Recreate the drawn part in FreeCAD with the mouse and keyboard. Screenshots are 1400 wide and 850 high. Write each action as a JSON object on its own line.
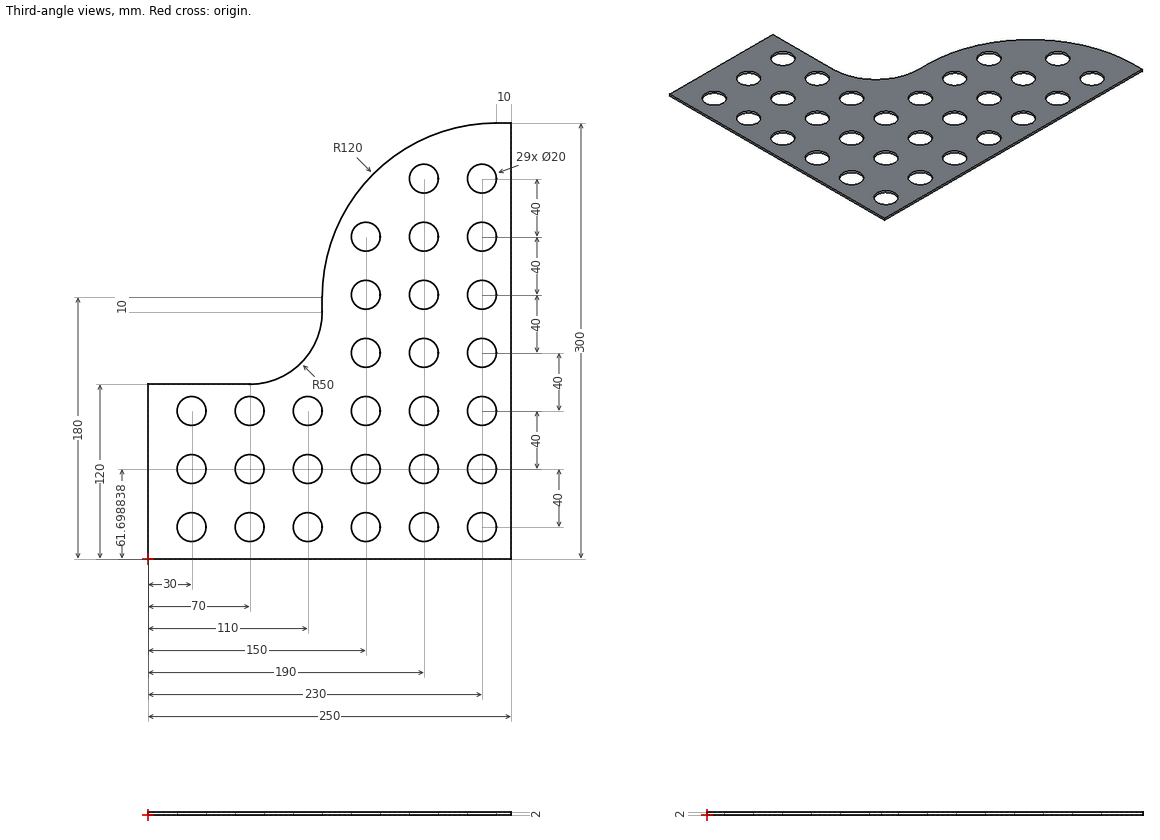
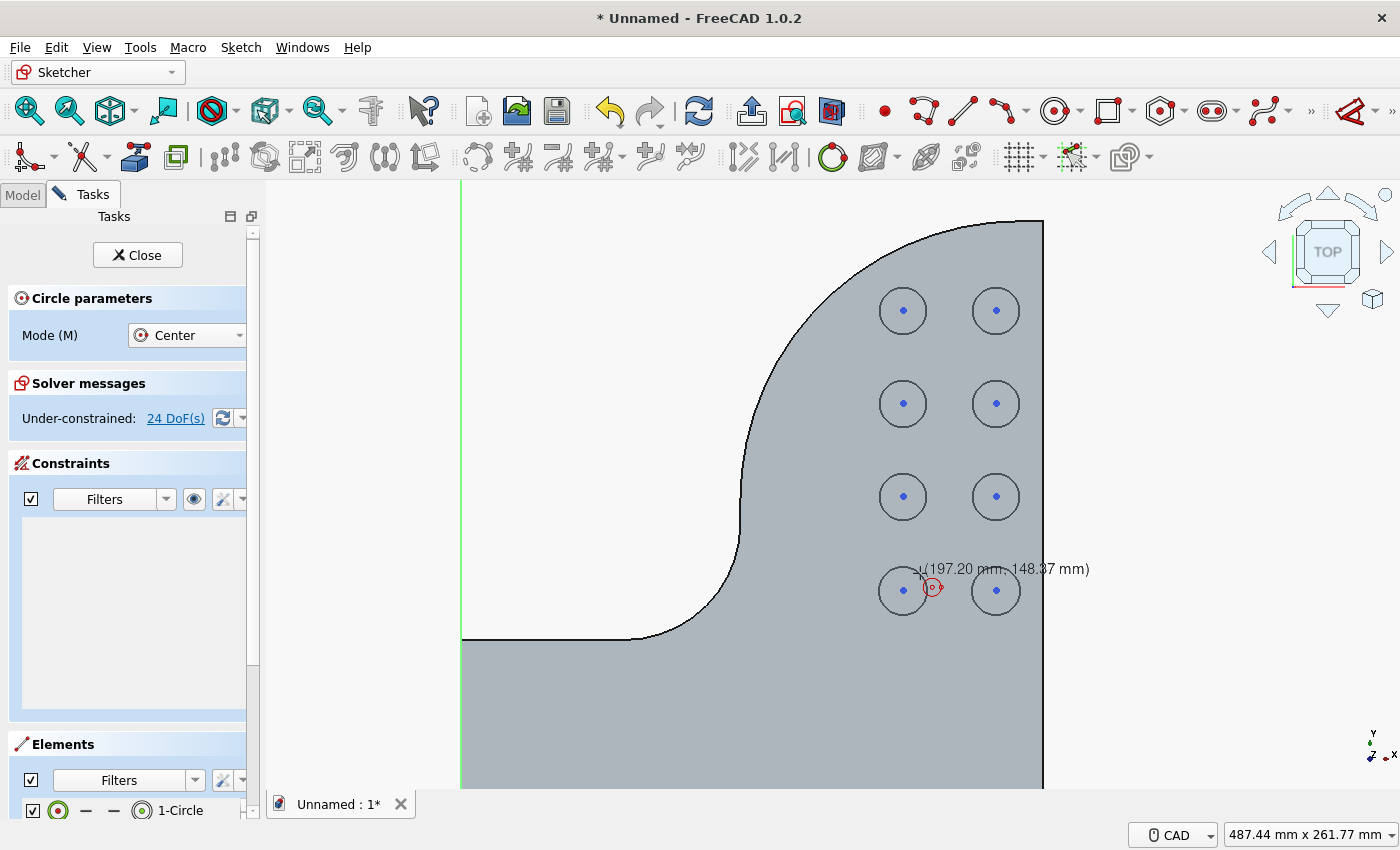
{"action": "left_click", "coordinate": [996, 683]}
{"action": "left_click", "coordinate": [1013, 666]}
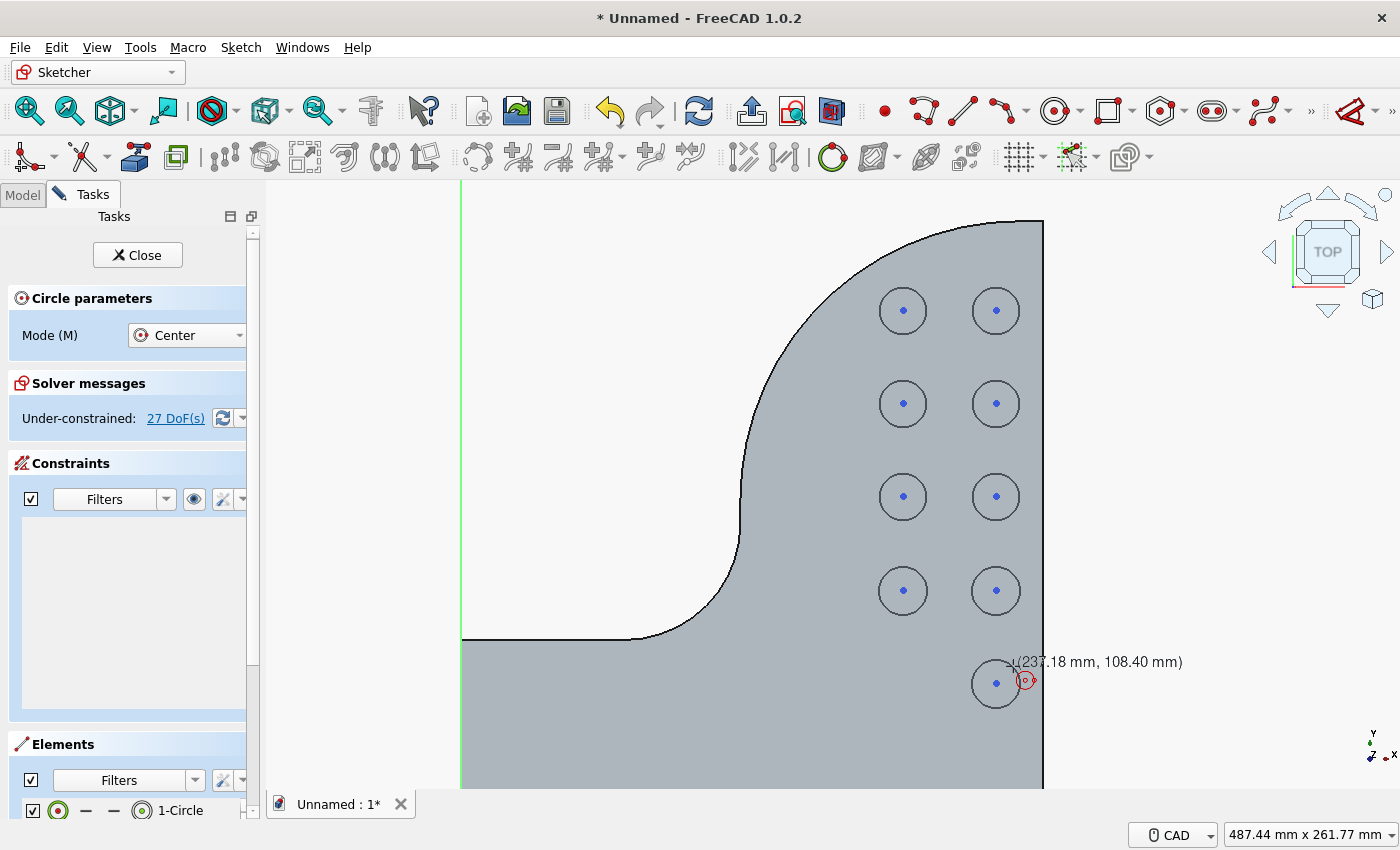
{"action": "left_click", "coordinate": [903, 683]}
{"action": "left_click", "coordinate": [920, 666]}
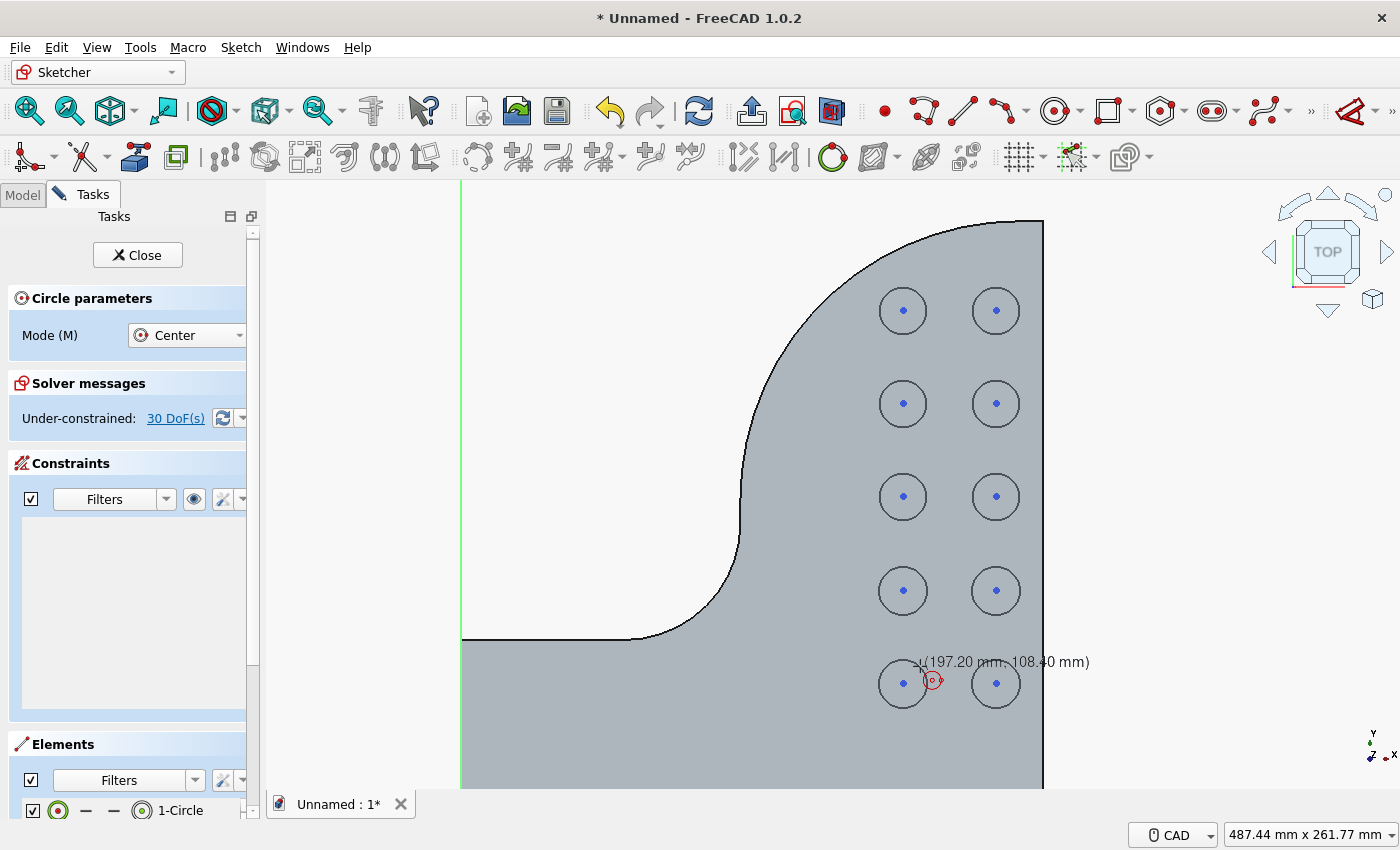
{"action": "scroll", "coordinate": [814, 243], "scroll_direction": "down", "scroll_amount": 2}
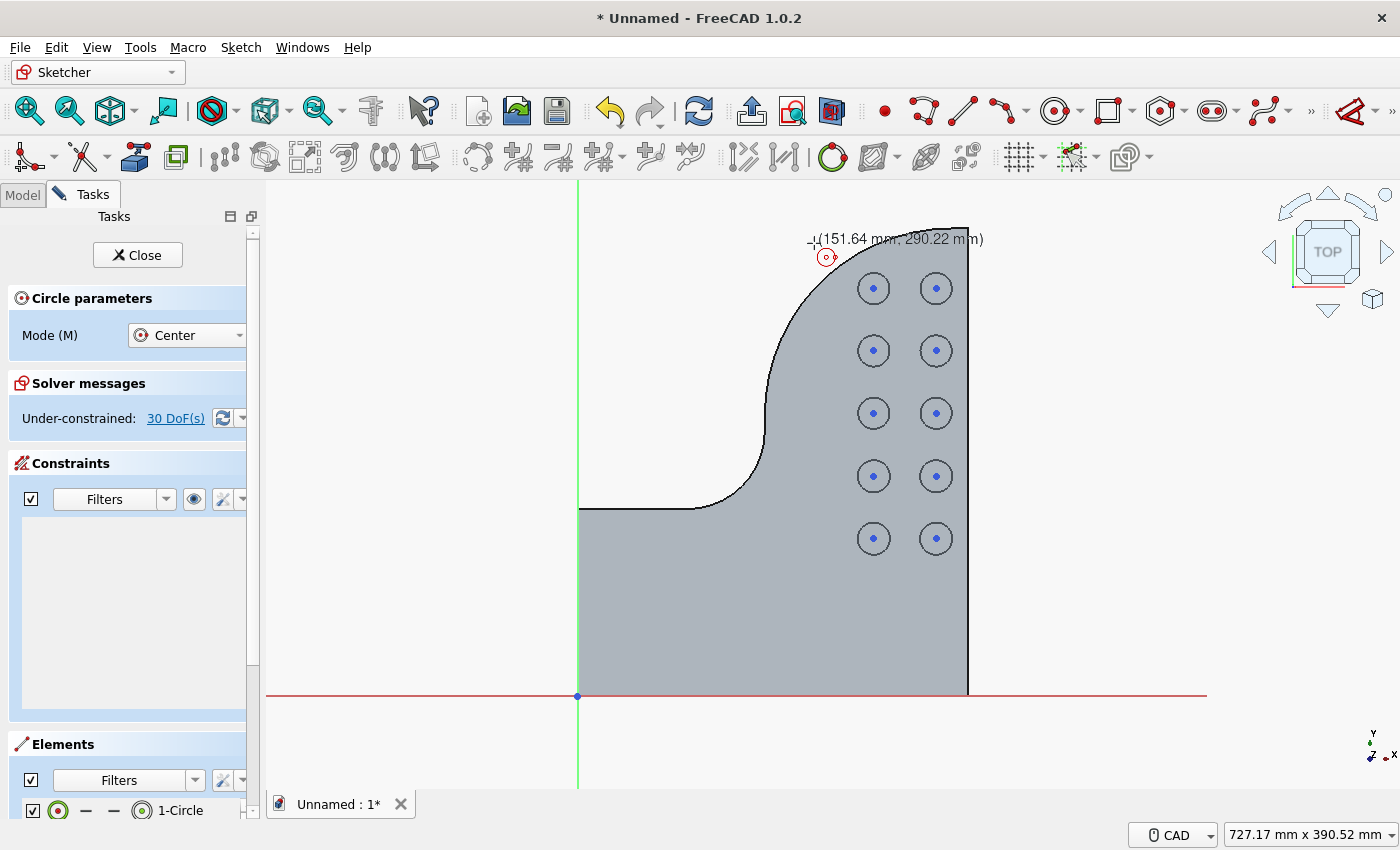
{"action": "scroll", "coordinate": [936, 600], "scroll_direction": "up", "scroll_amount": 2}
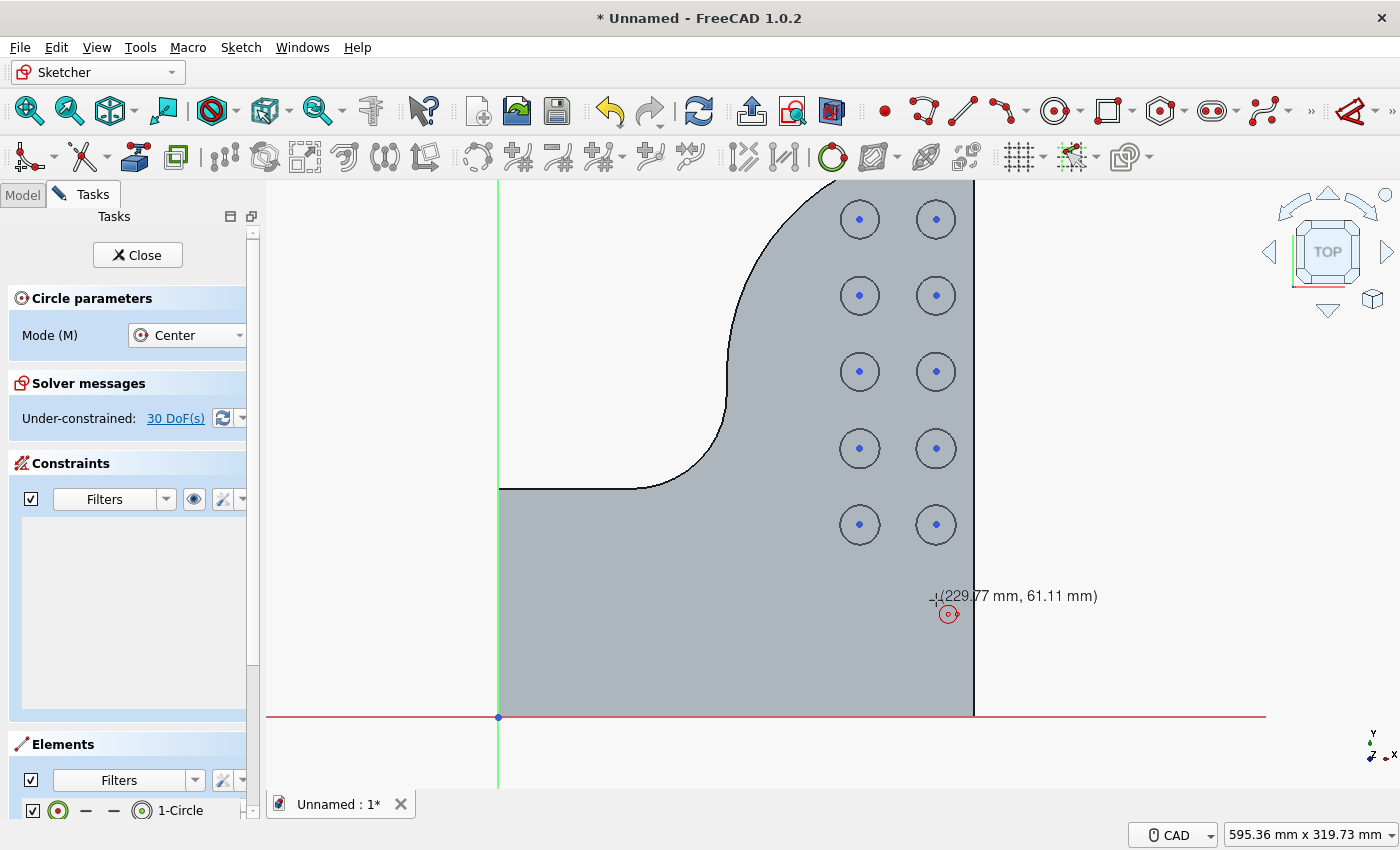
{"action": "left_click", "coordinate": [936, 600]}
{"action": "left_click", "coordinate": [953, 583]}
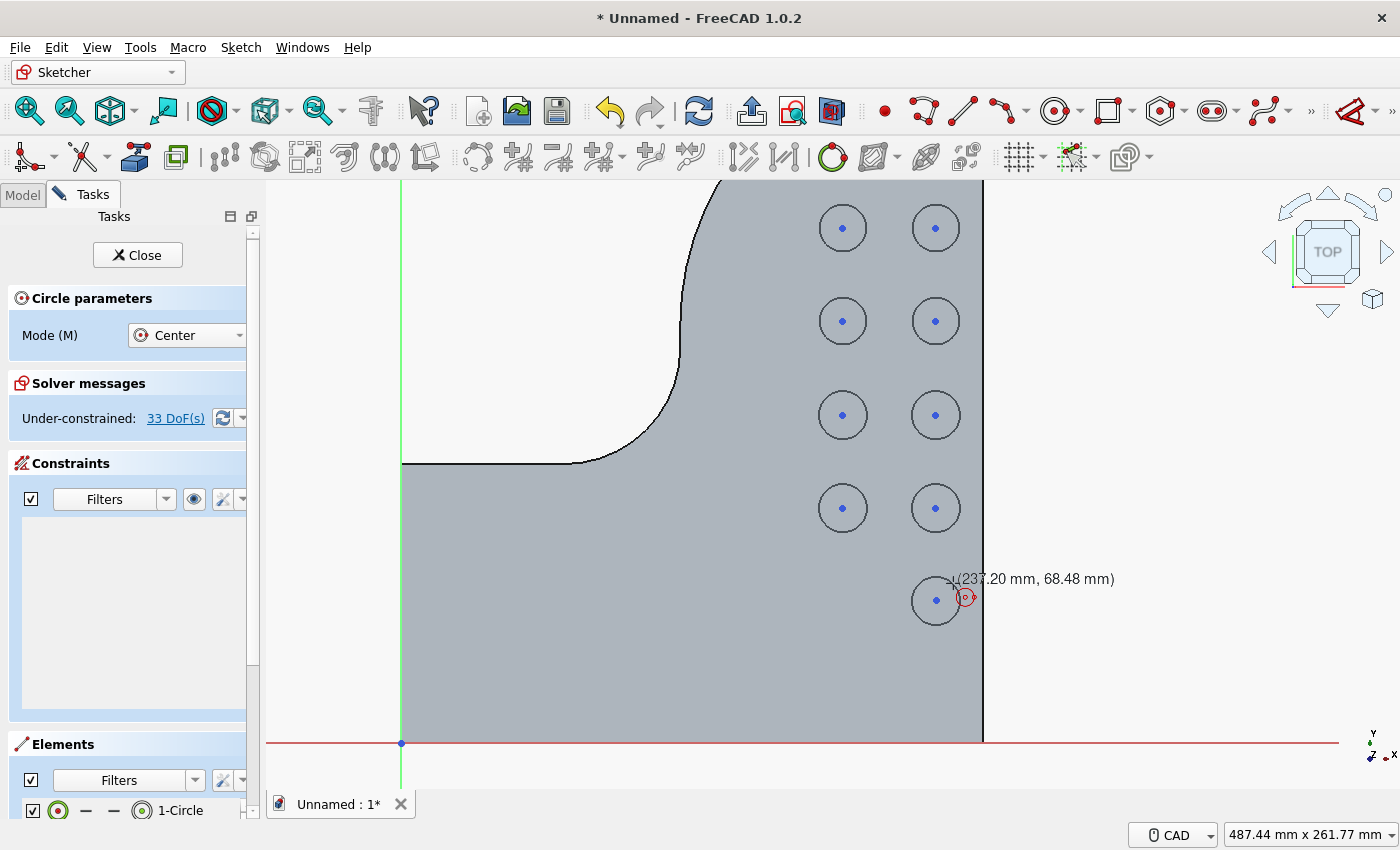
{"action": "left_click", "coordinate": [843, 600]}
{"action": "left_click", "coordinate": [860, 583]}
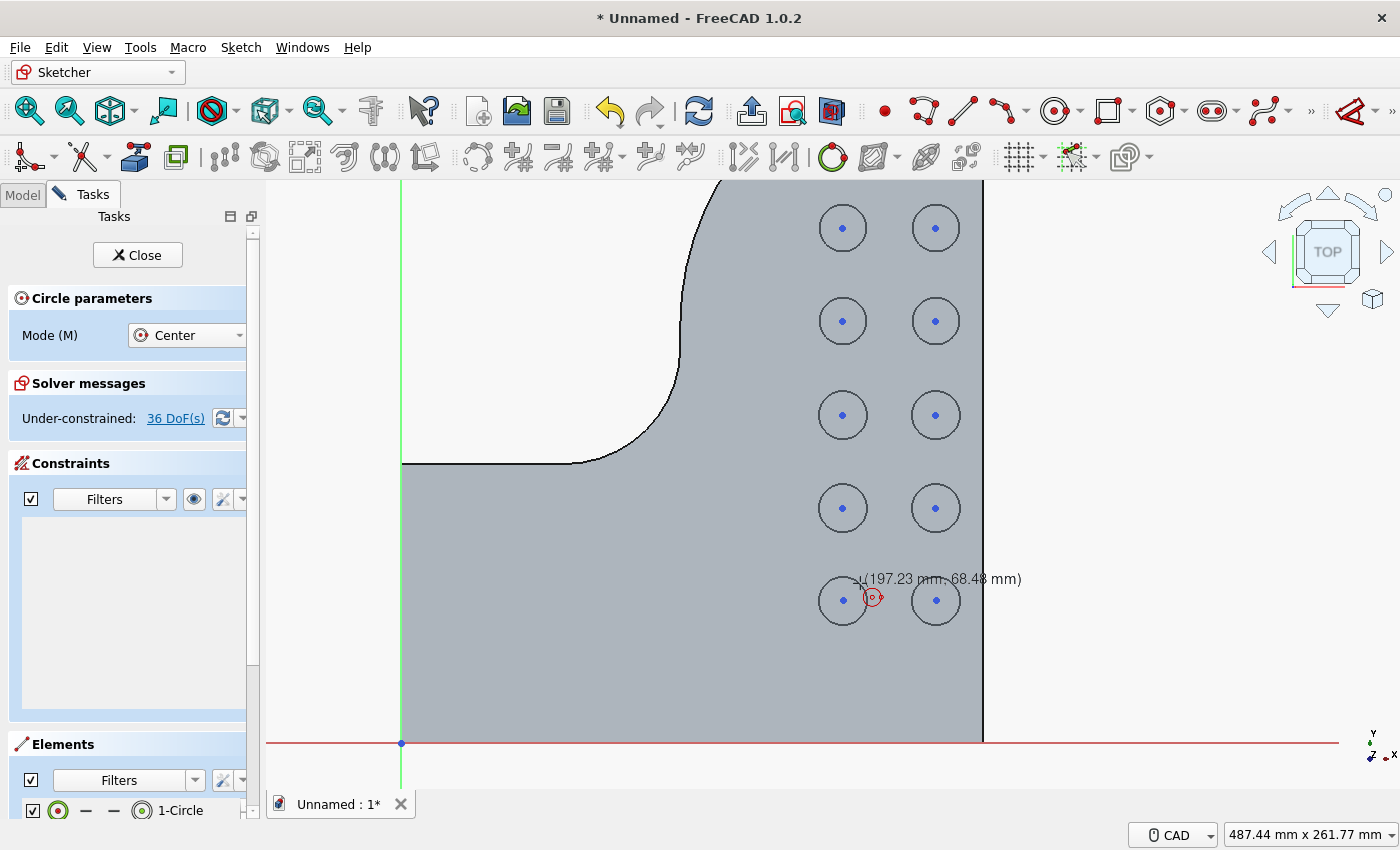
{"action": "left_click", "coordinate": [936, 693]}
{"action": "left_click", "coordinate": [953, 676]}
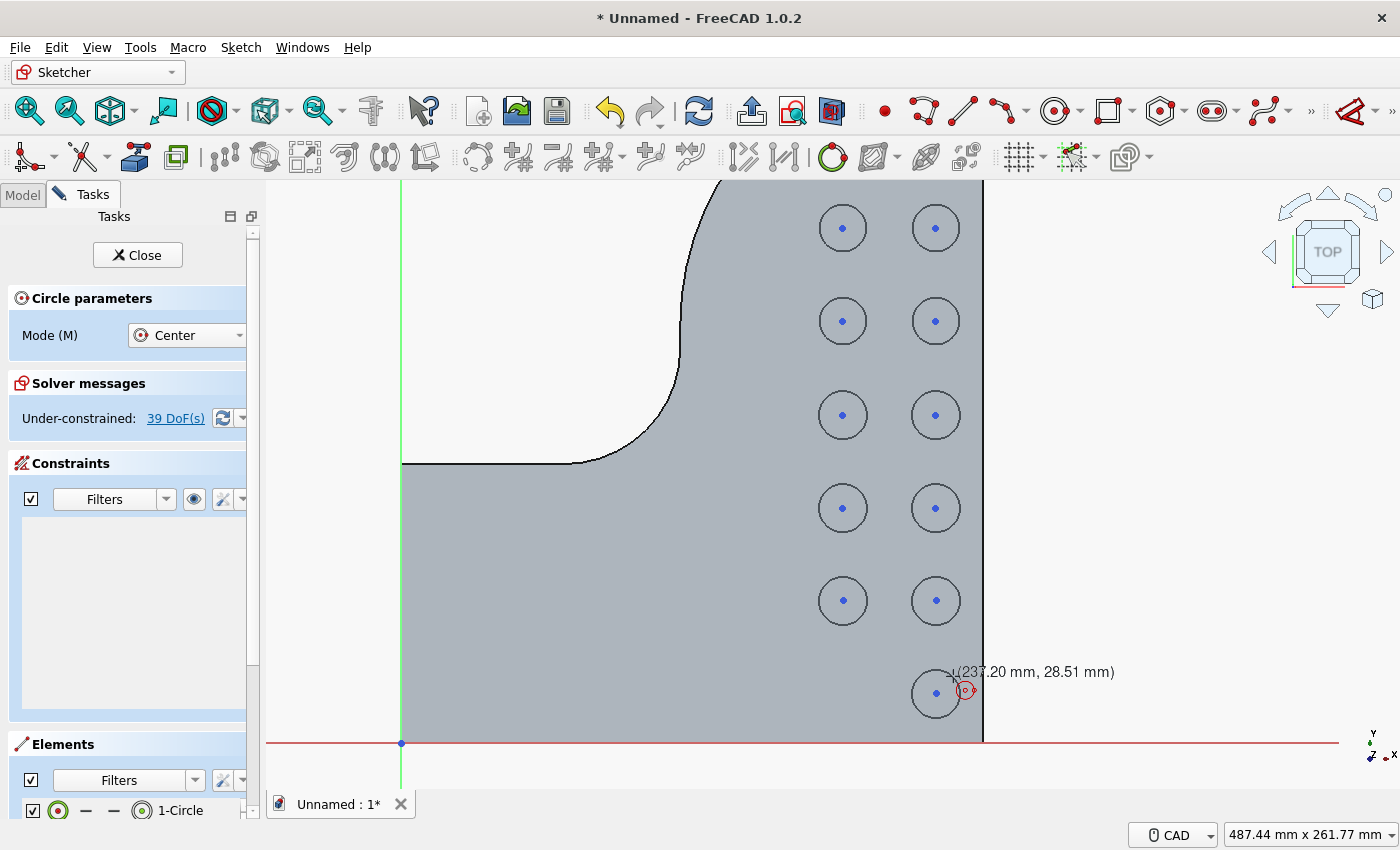
{"action": "left_click", "coordinate": [843, 693]}
{"action": "left_click", "coordinate": [860, 676]}